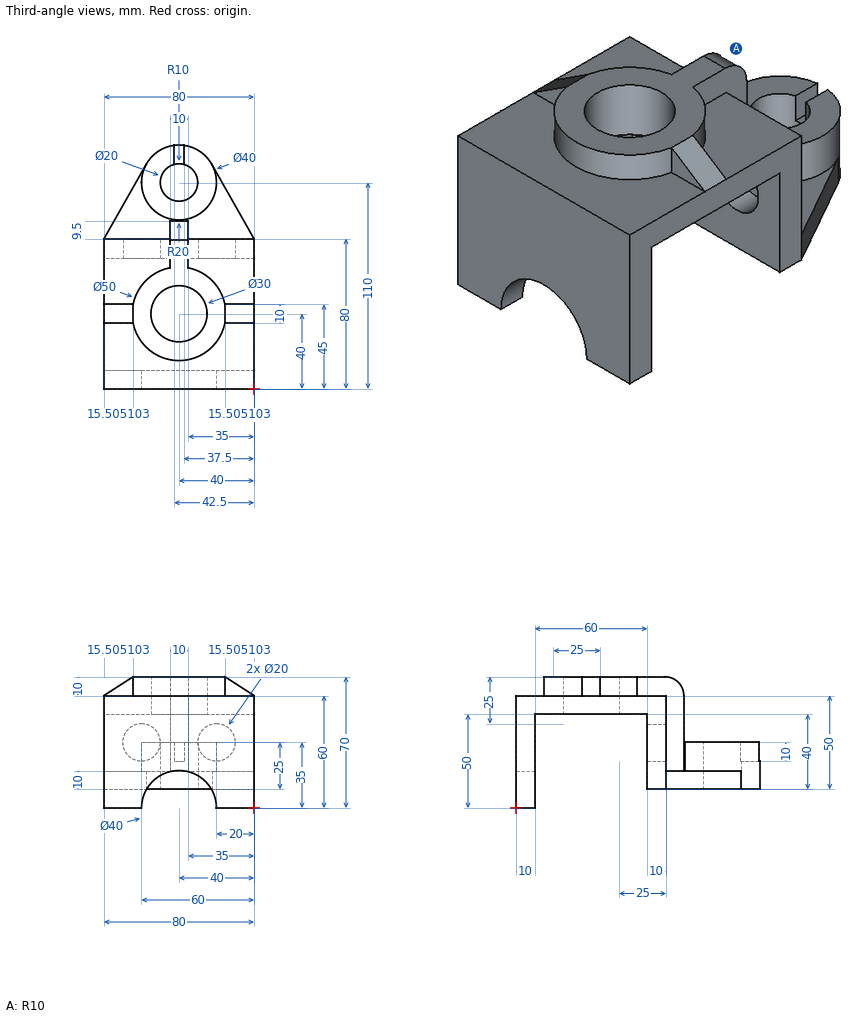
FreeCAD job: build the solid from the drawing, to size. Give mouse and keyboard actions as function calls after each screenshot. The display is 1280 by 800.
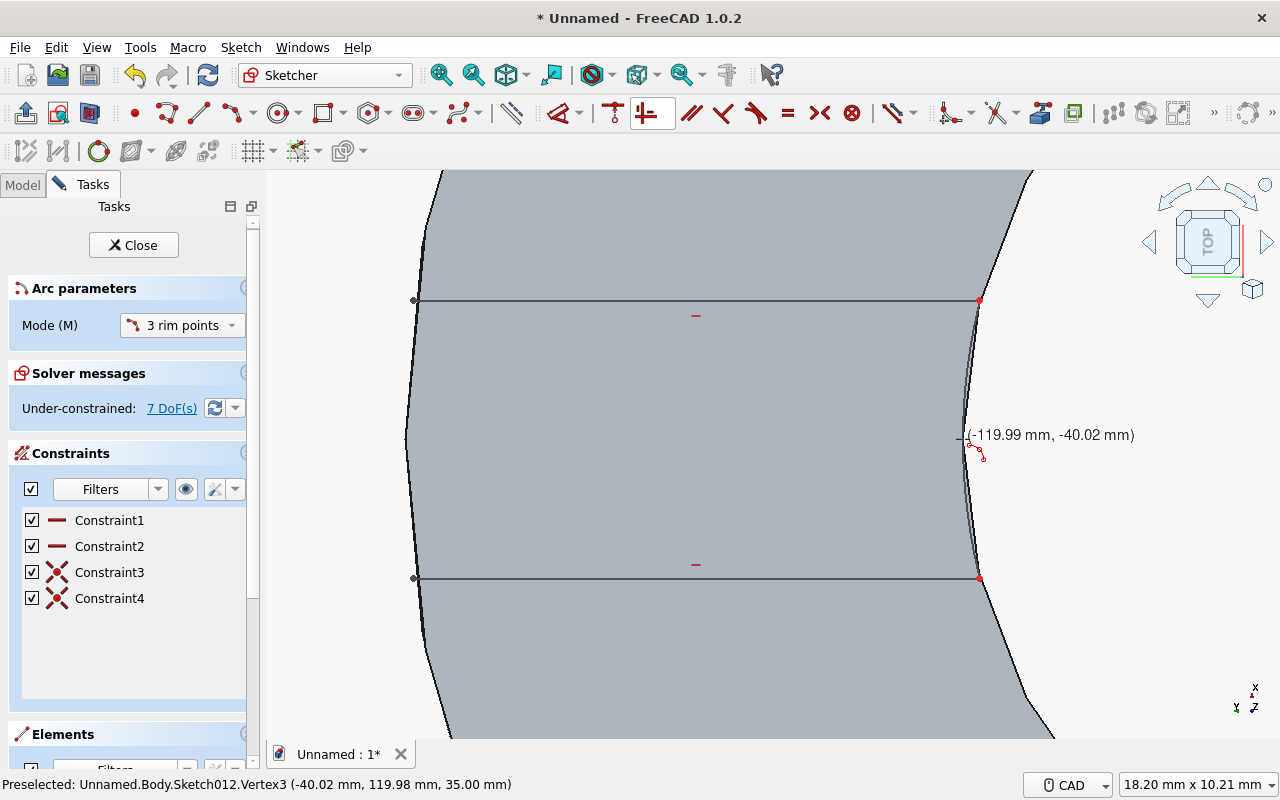
click(414, 301)
click(414, 579)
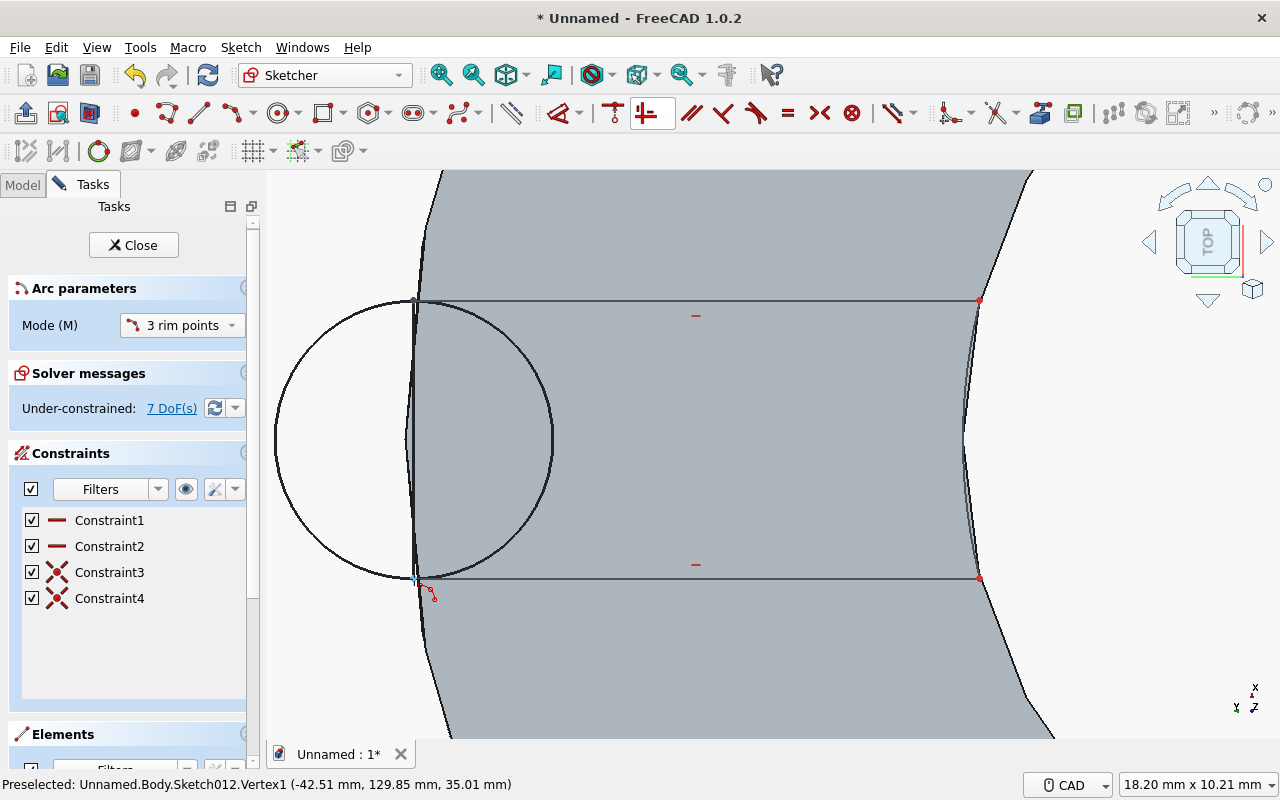
scroll(405, 439, up, 3)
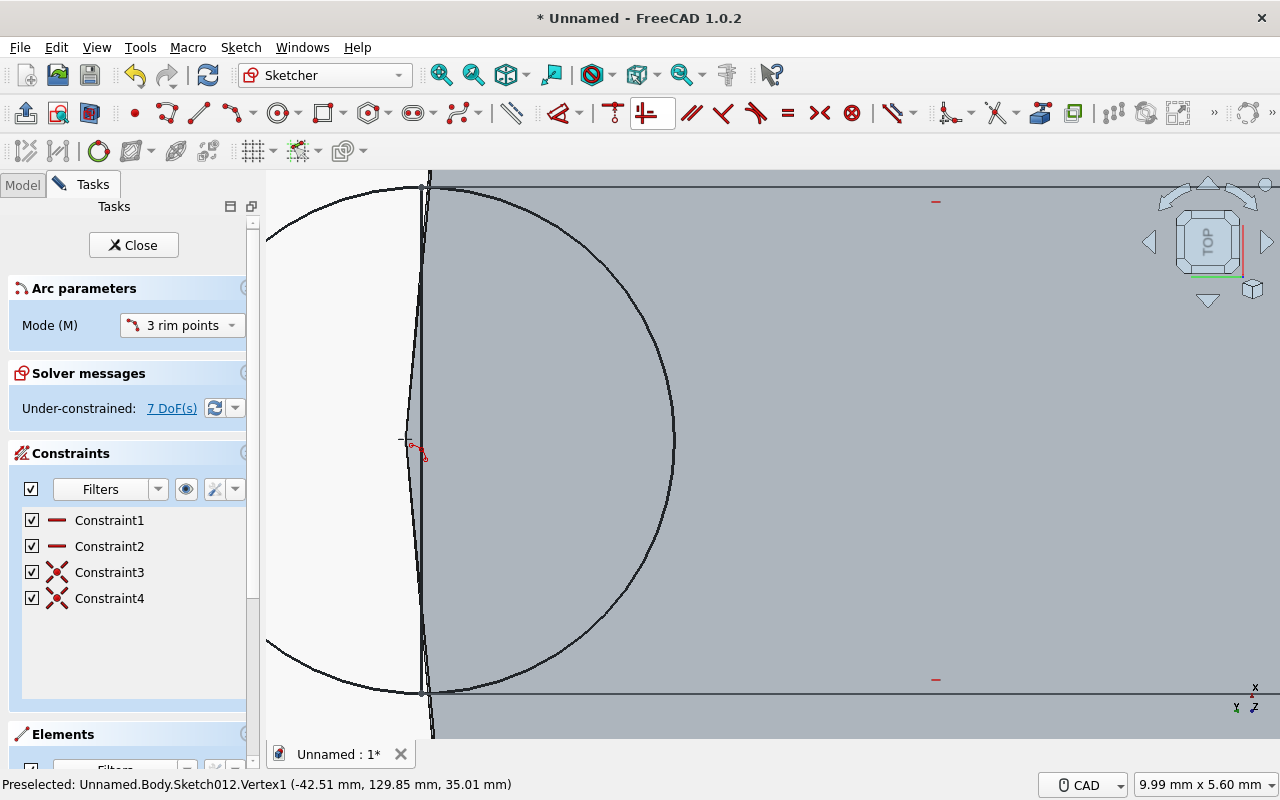
click(406, 439)
key(Escape)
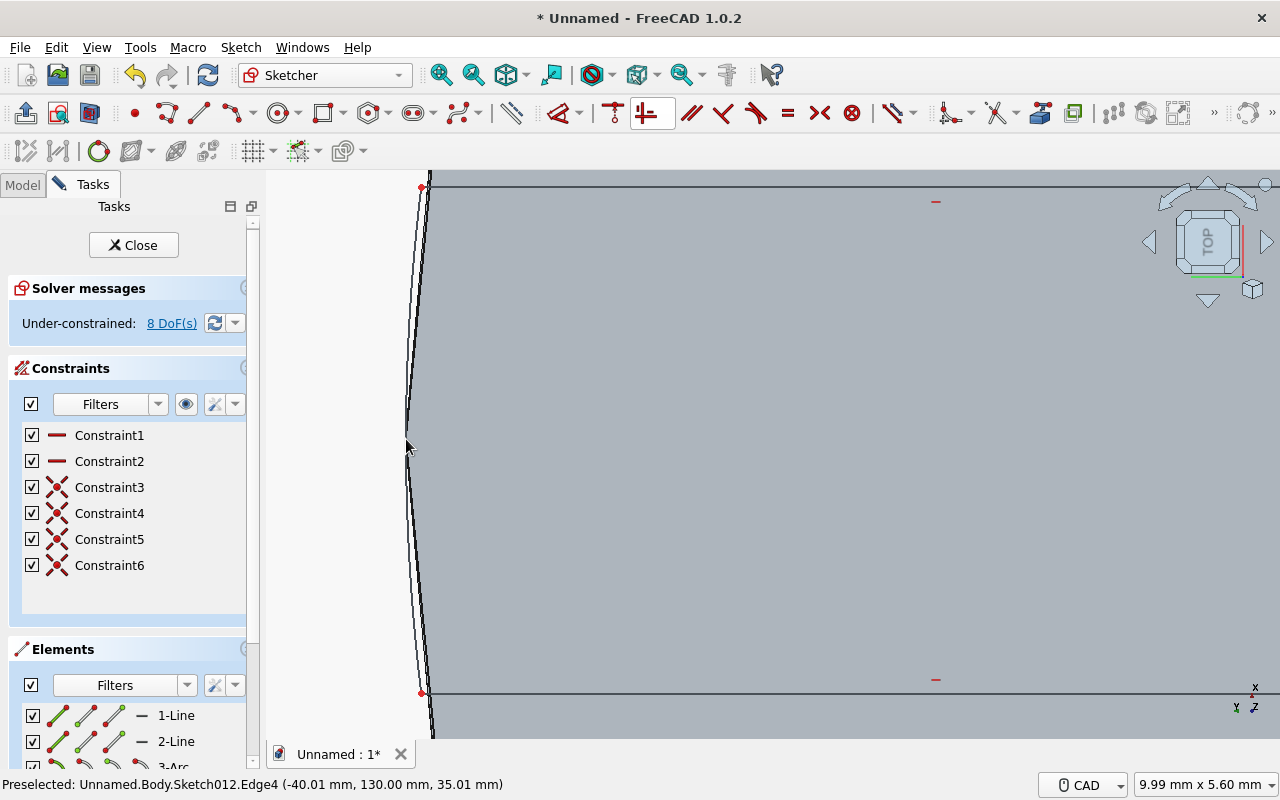
scroll(431, 474, down, 3)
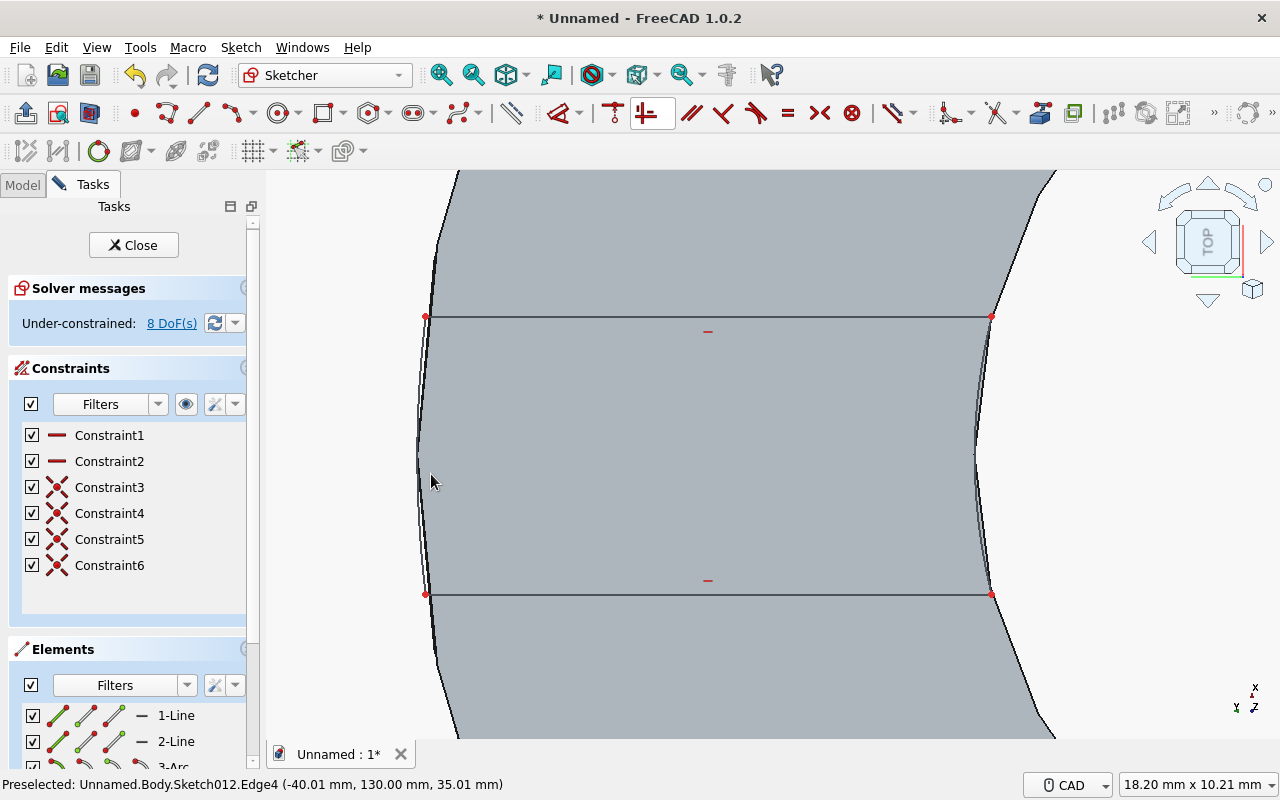
click(977, 400)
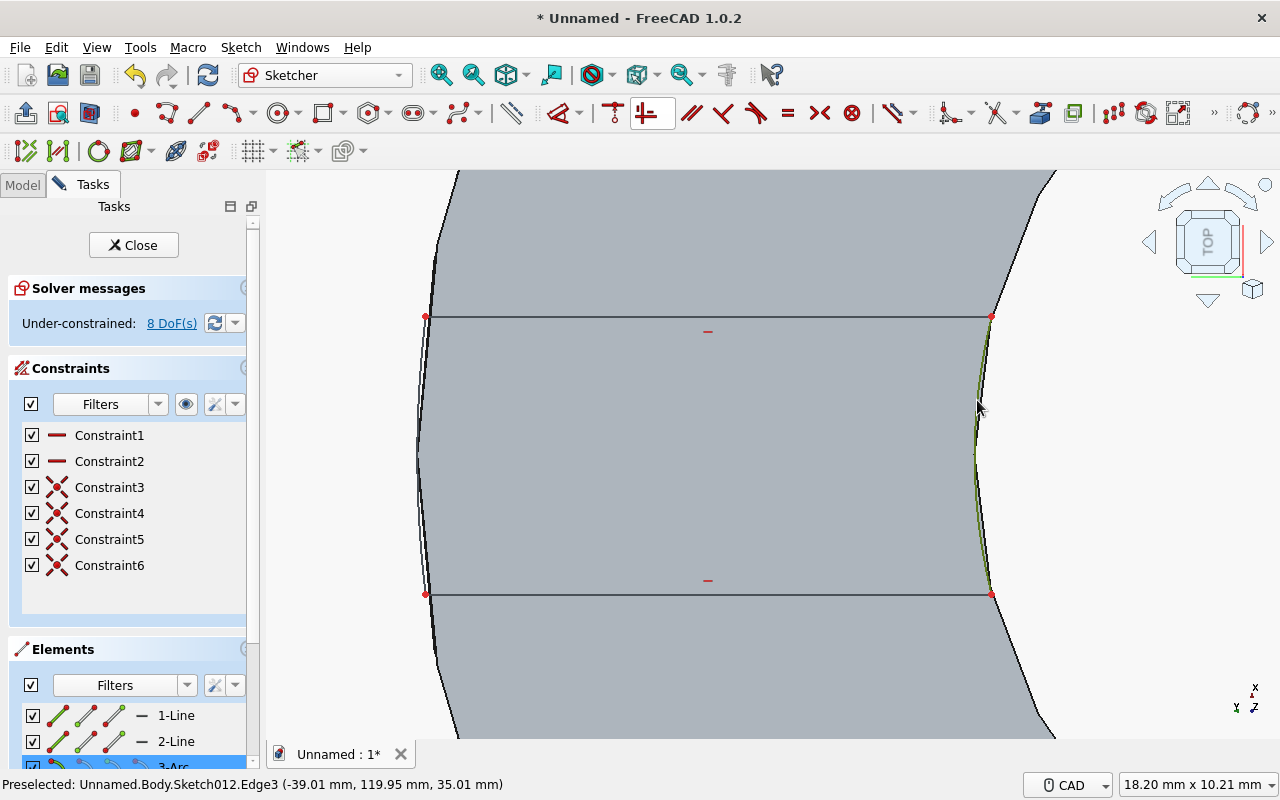
click(419, 400)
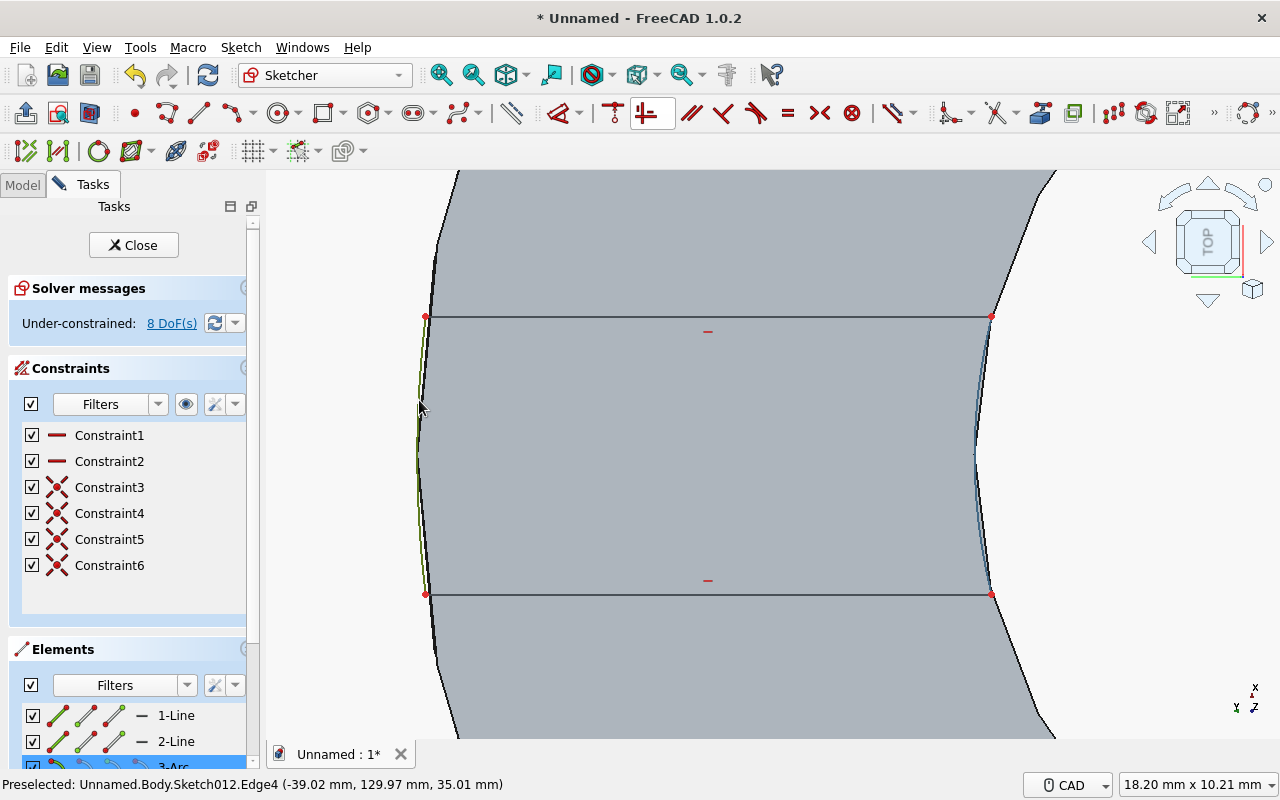
click(614, 114)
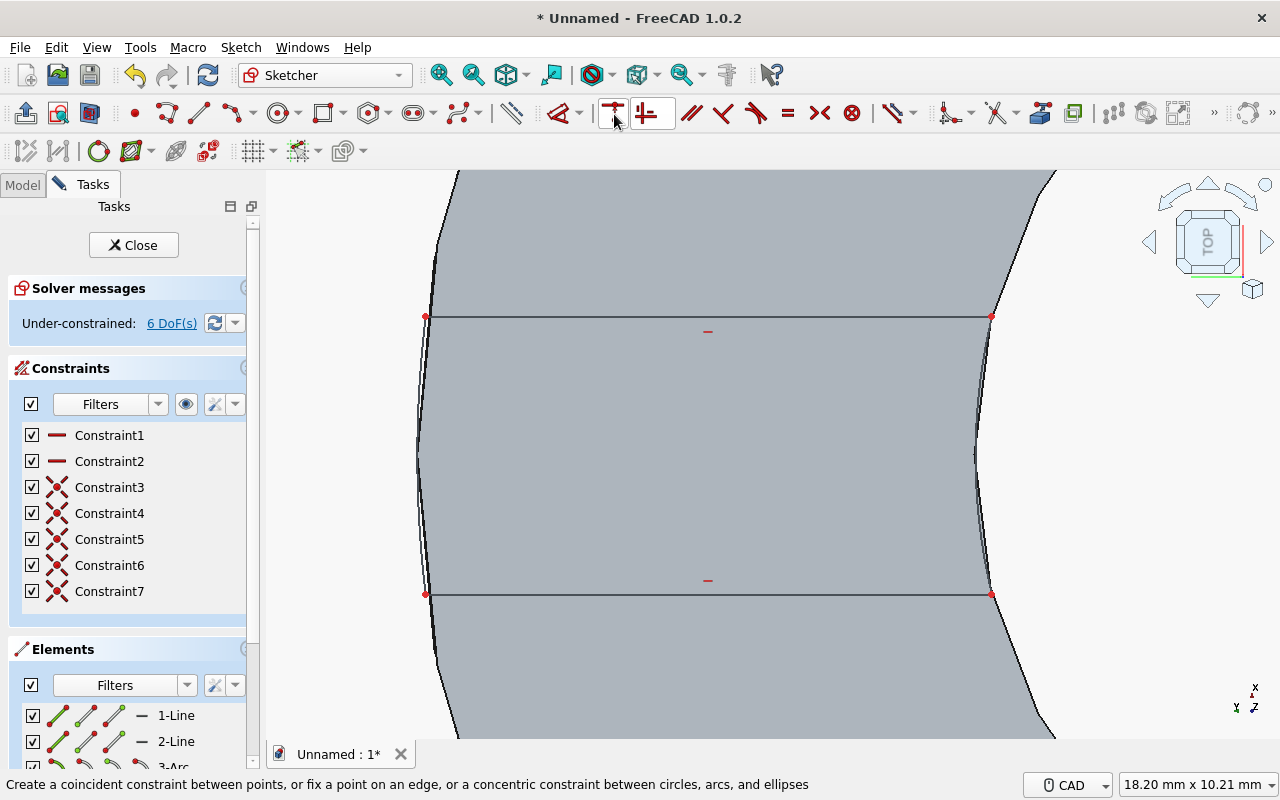
click(558, 114)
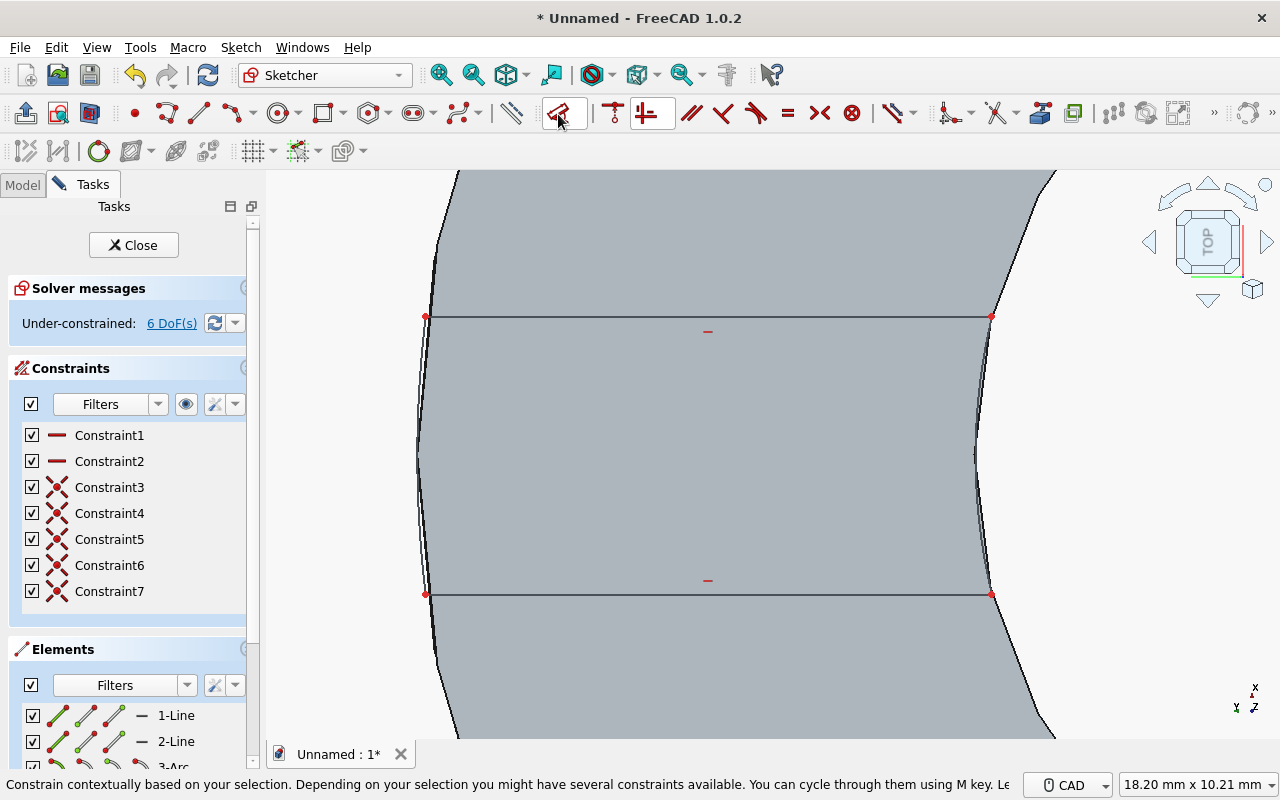
click(978, 400)
click(946, 397)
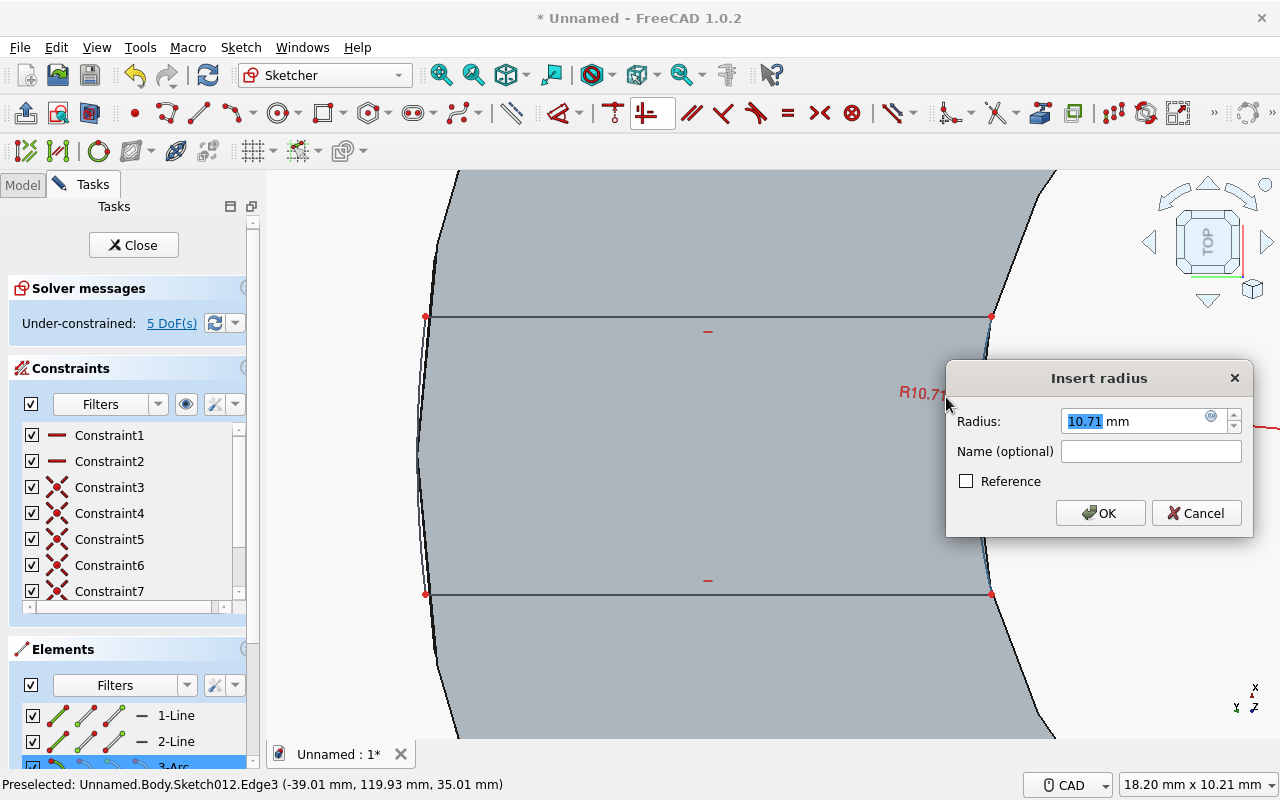
text(10)
key(Return)